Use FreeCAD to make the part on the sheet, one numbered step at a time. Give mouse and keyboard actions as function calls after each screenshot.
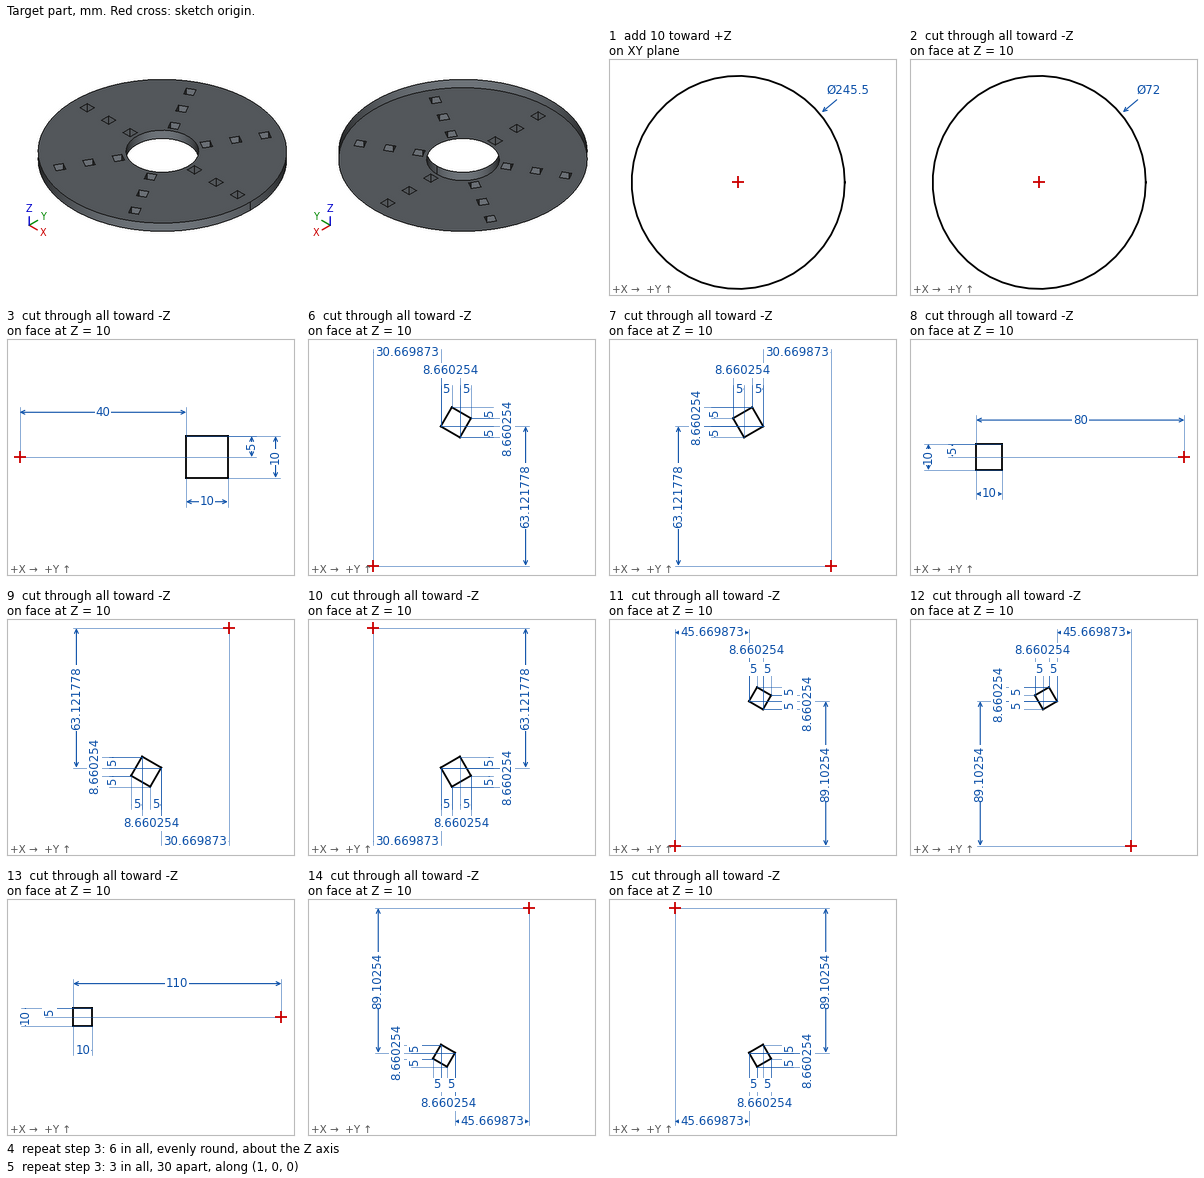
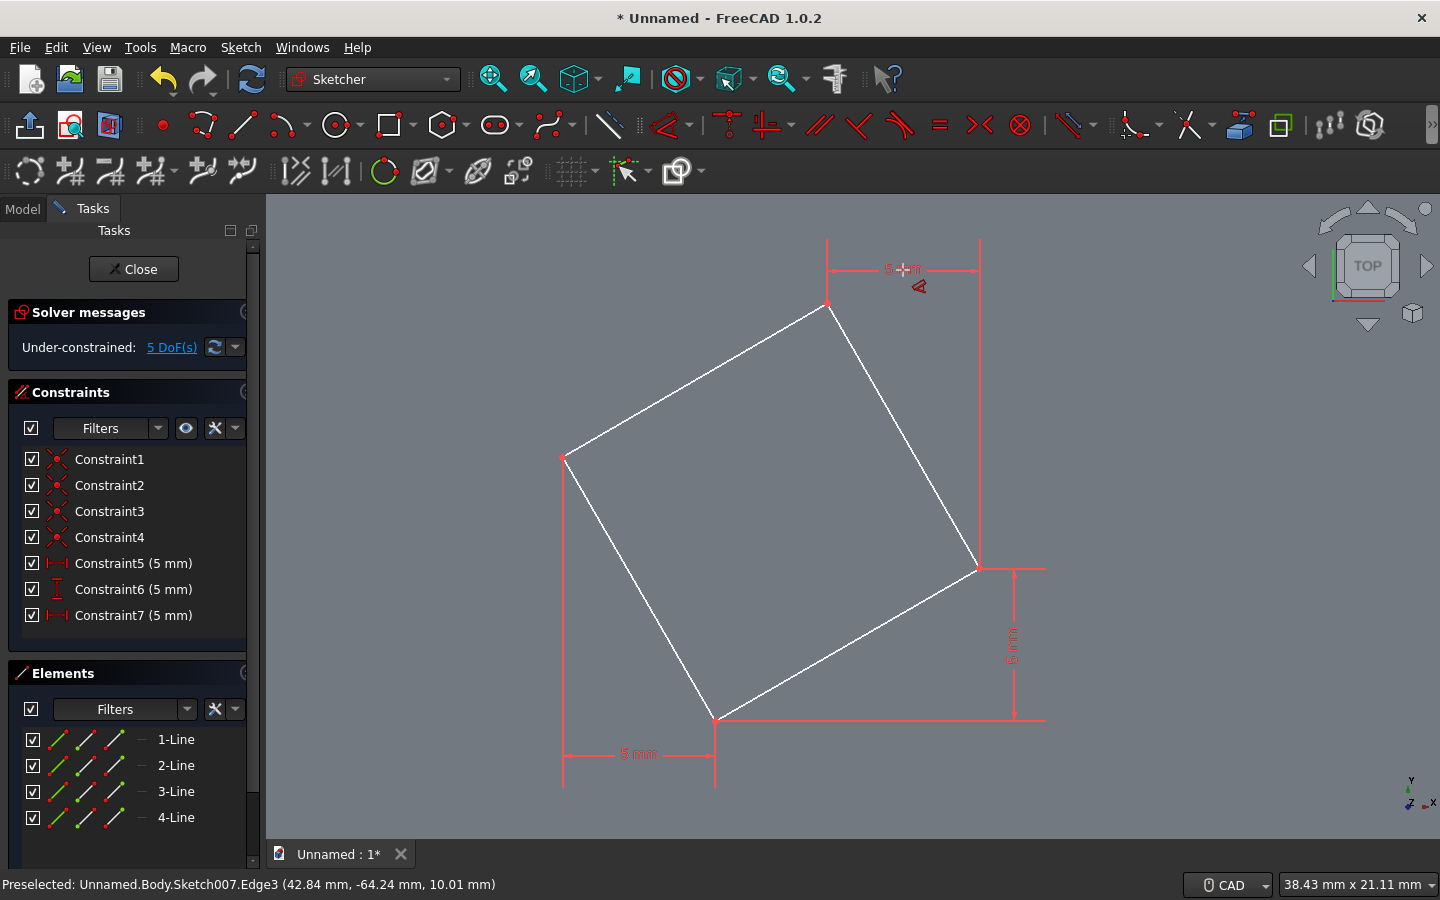
click(748, 350)
click(529, 380)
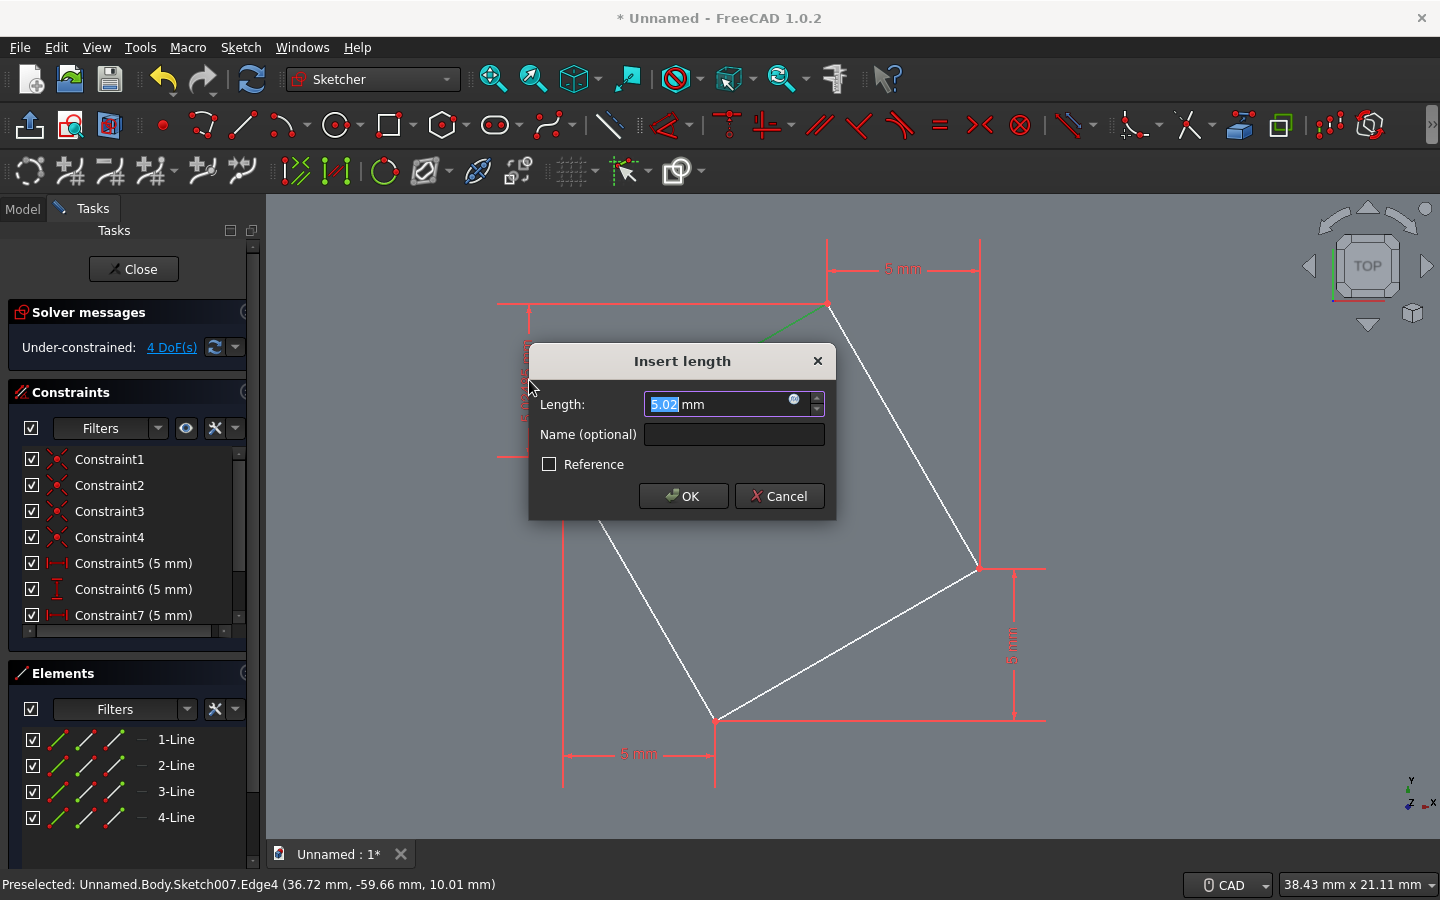
text(5)
key(Return)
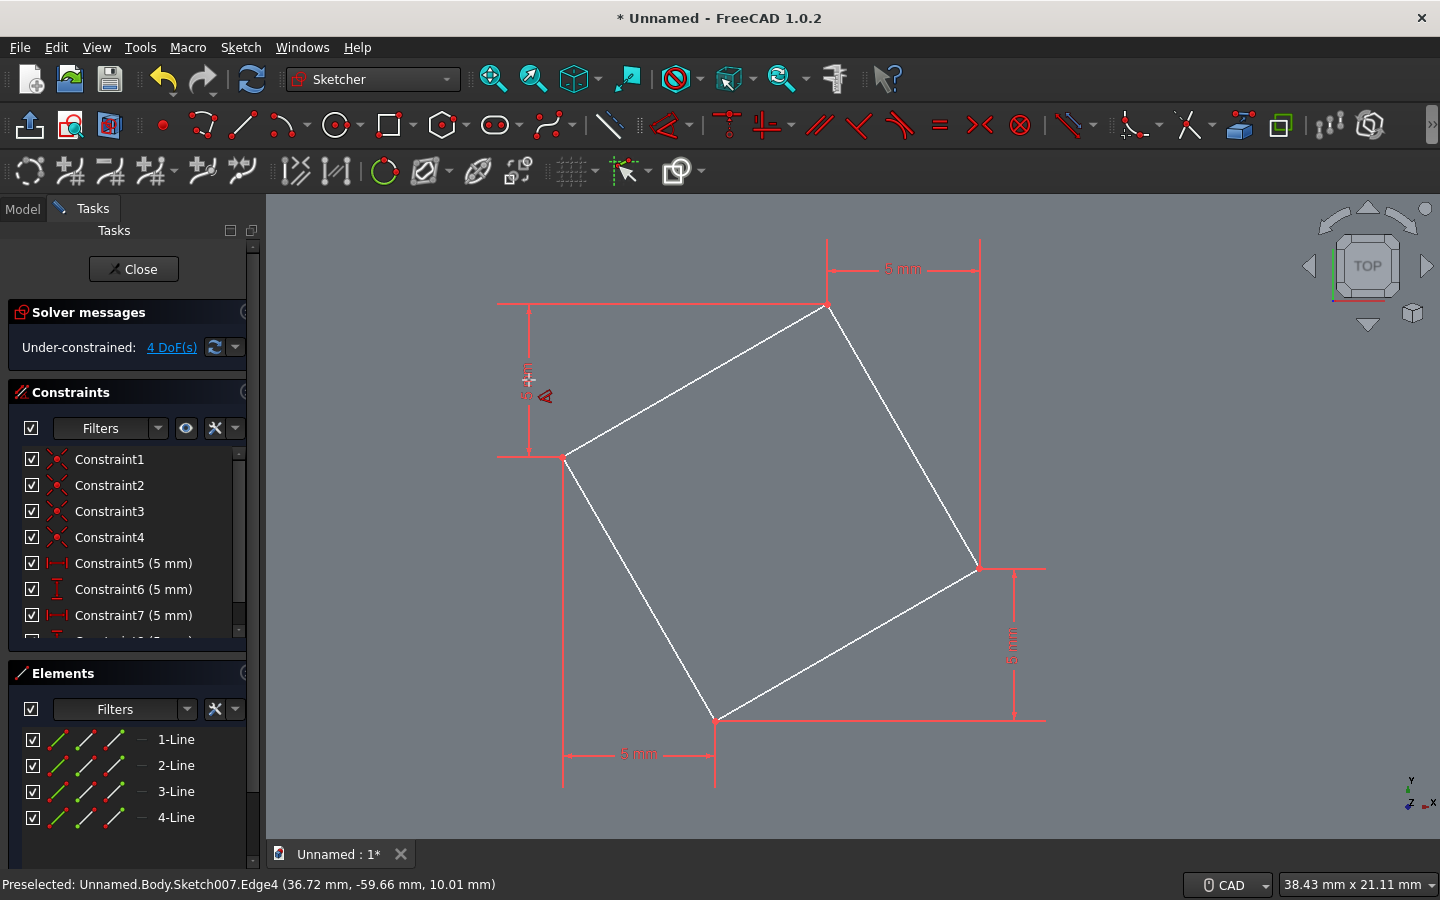
click(608, 536)
click(529, 589)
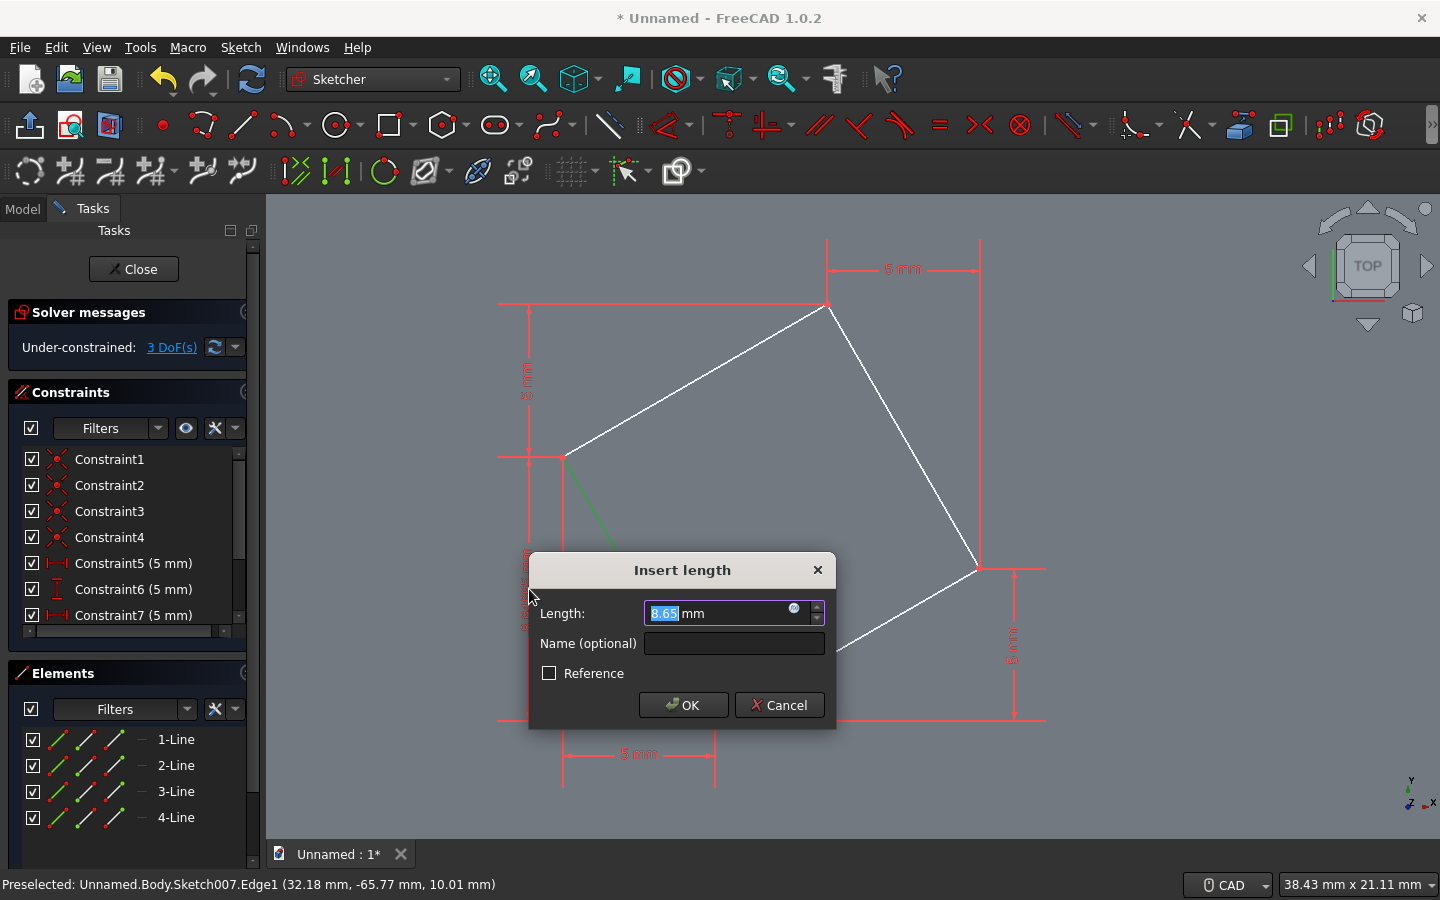
text(8.660254)
key(Return)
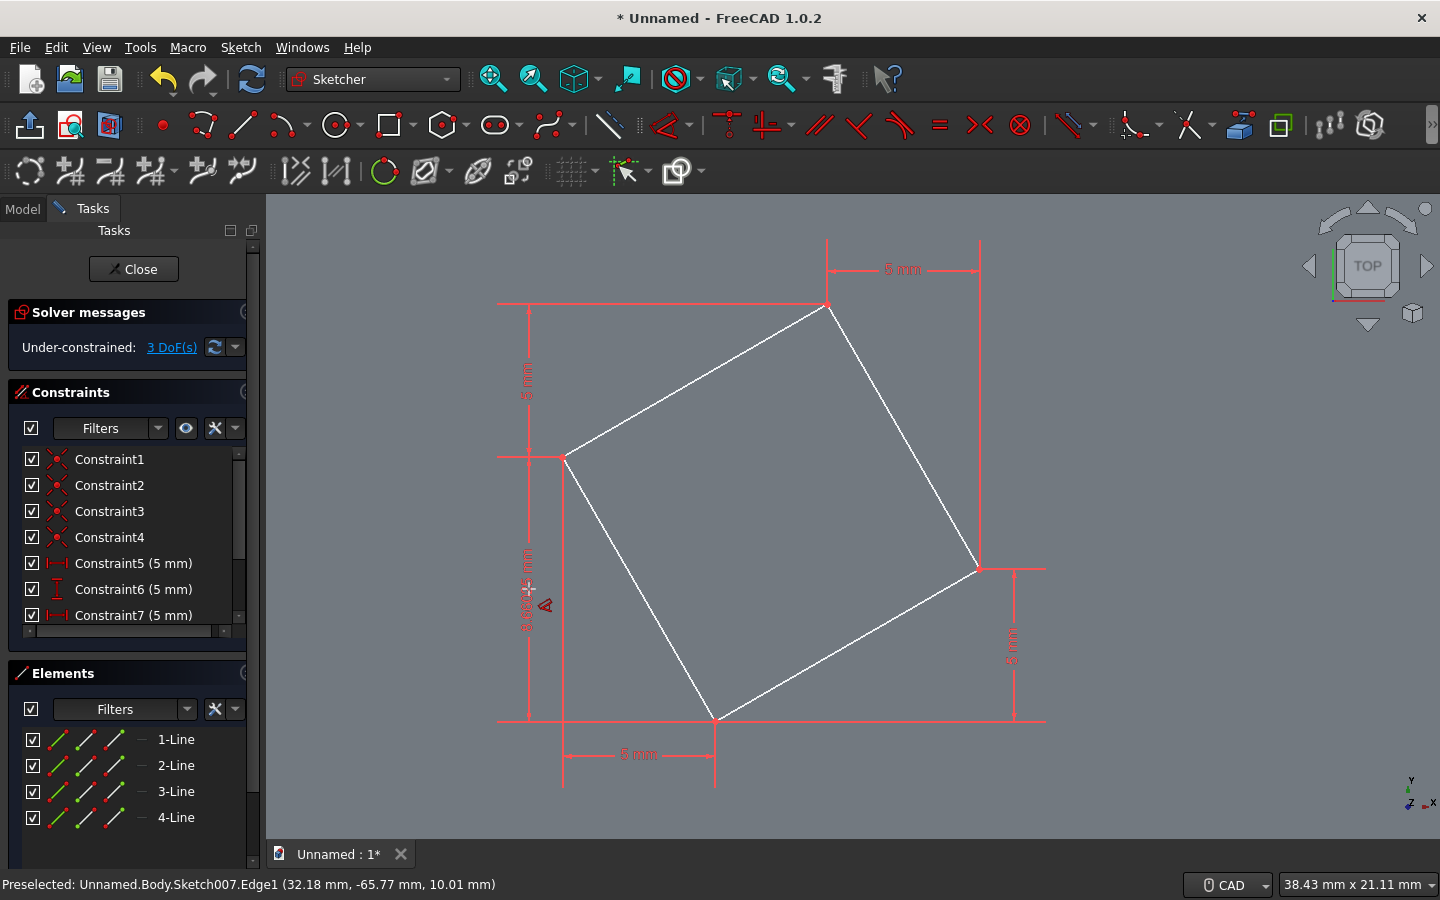
click(795, 676)
click(848, 756)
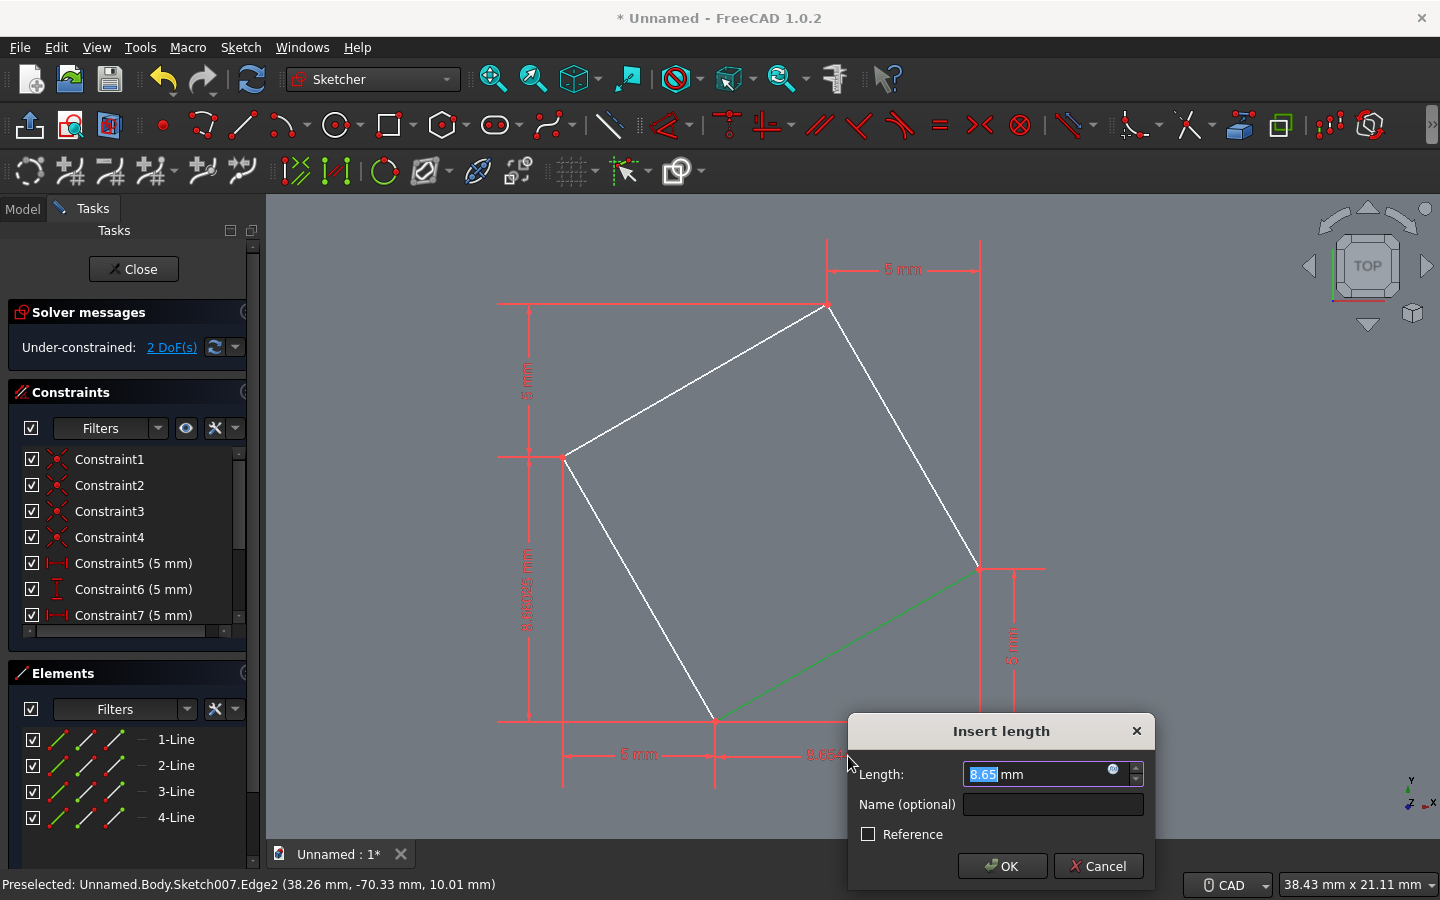
text(8.660254)
key(Return)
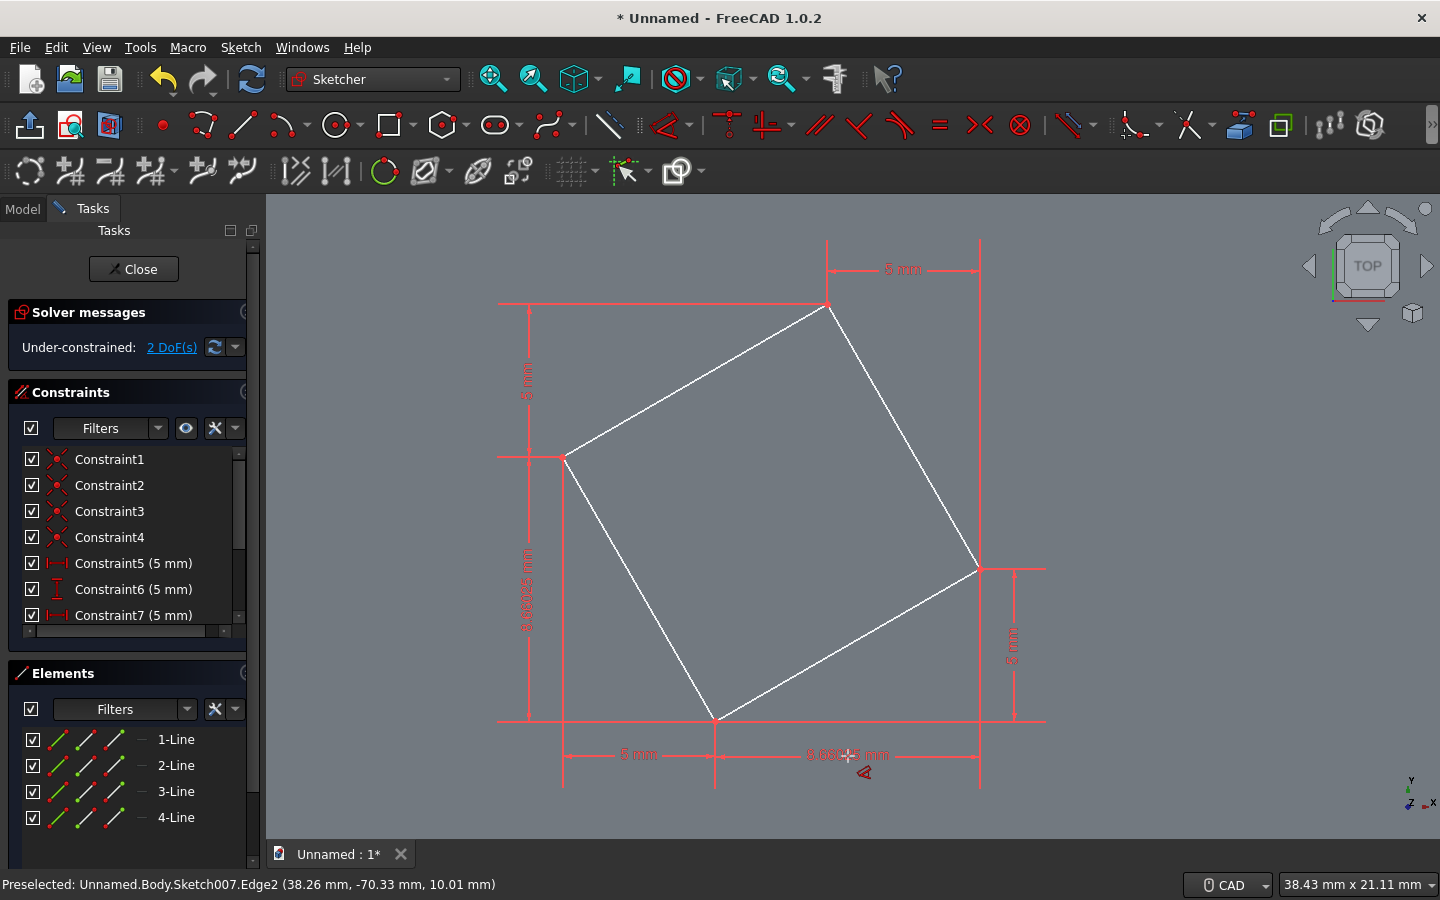
click(563, 457)
click(428, 491)